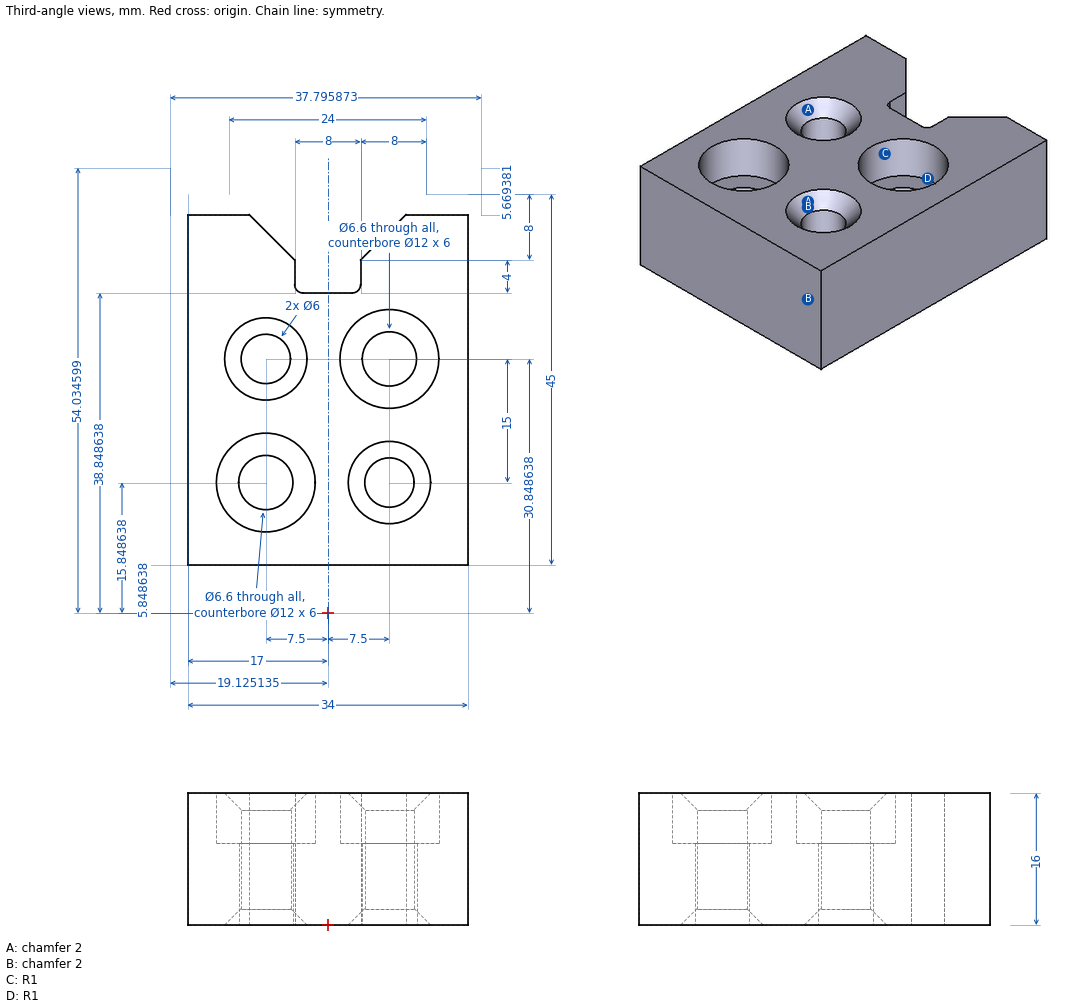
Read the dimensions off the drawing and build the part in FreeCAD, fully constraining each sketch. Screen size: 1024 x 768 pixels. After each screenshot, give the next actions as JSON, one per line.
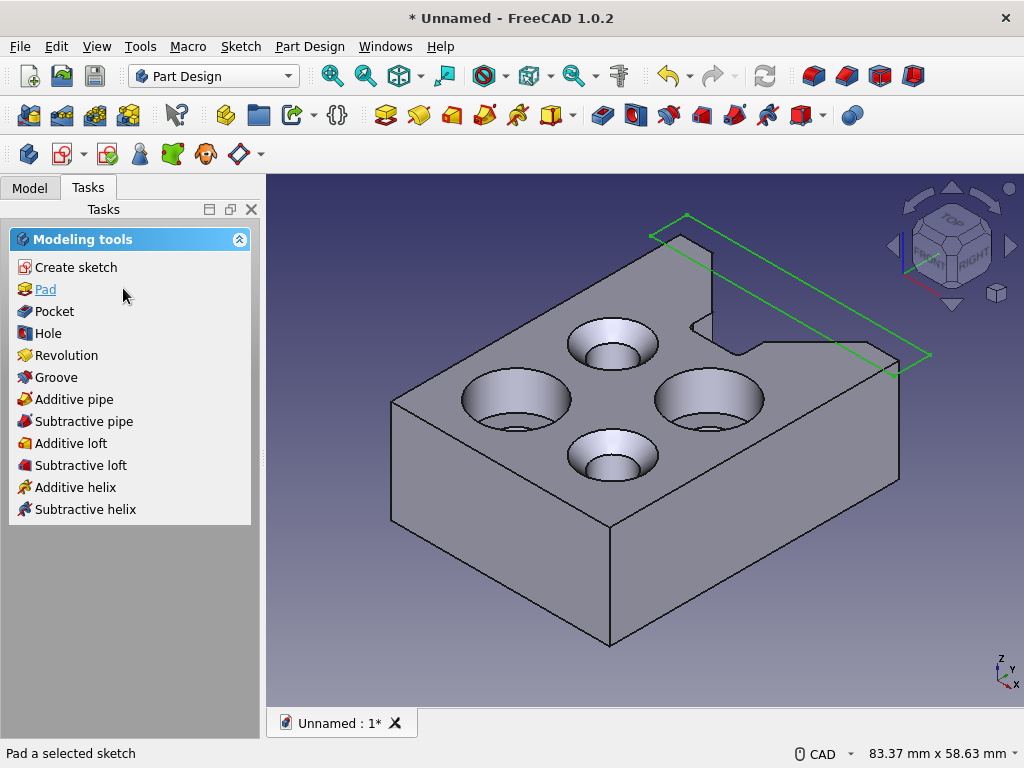
{"action": "left_click", "coordinate": [603, 116]}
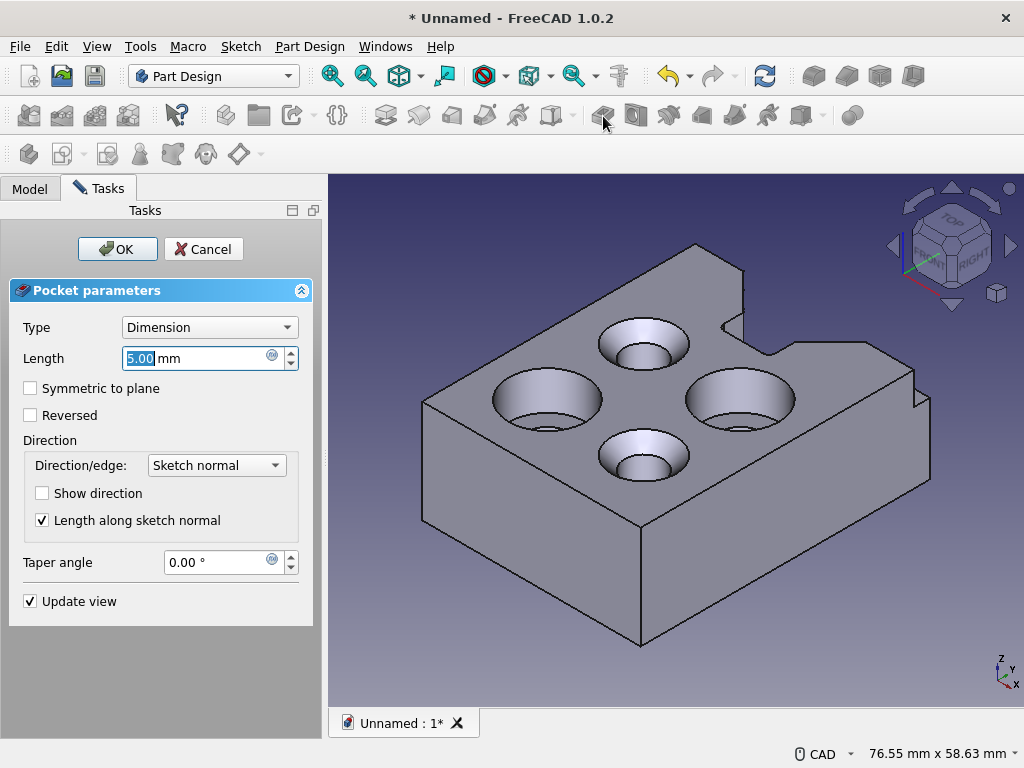
{"action": "left_click", "coordinate": [210, 328]}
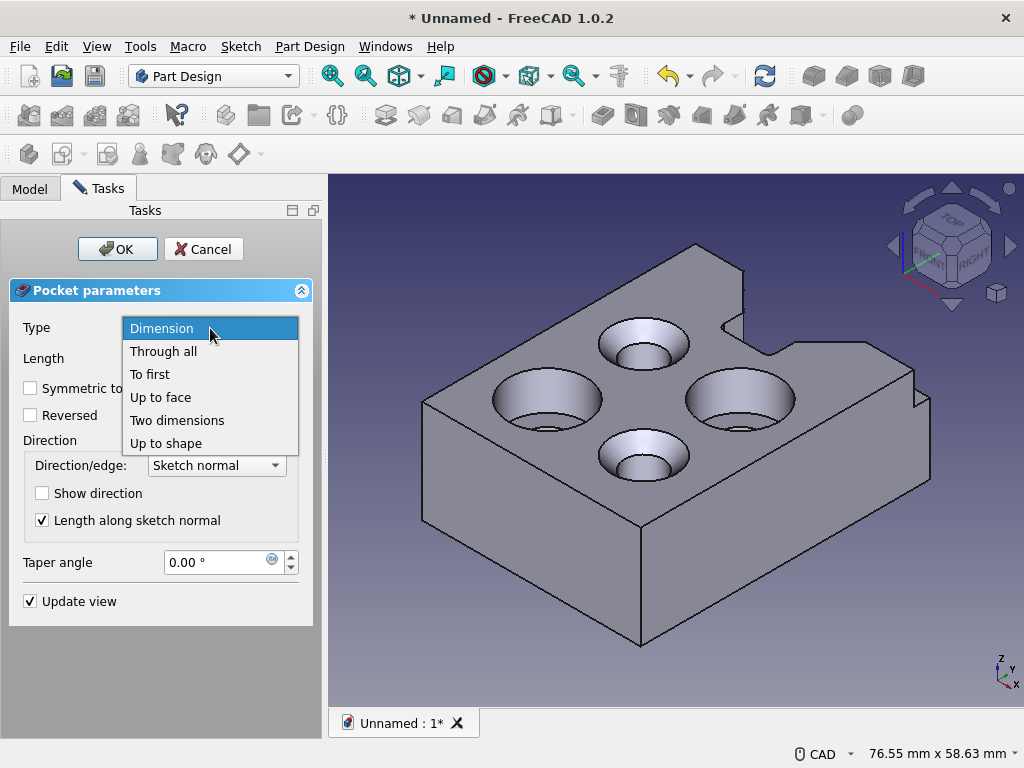
{"action": "left_click", "coordinate": [208, 352]}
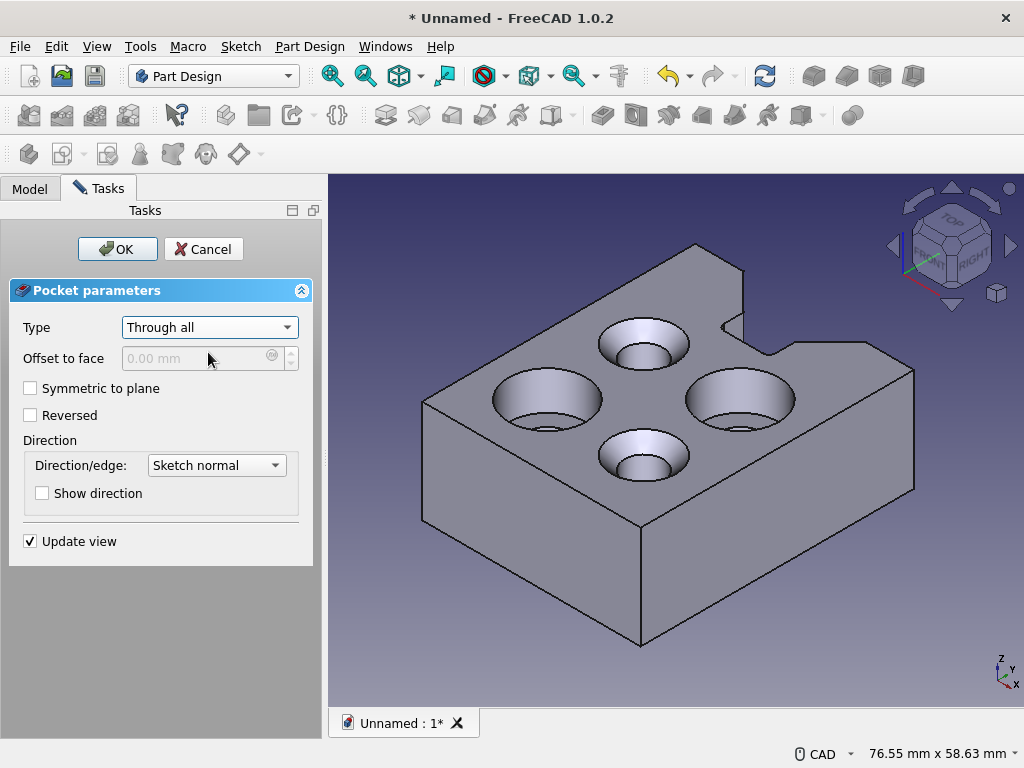
{"action": "left_click", "coordinate": [118, 249]}